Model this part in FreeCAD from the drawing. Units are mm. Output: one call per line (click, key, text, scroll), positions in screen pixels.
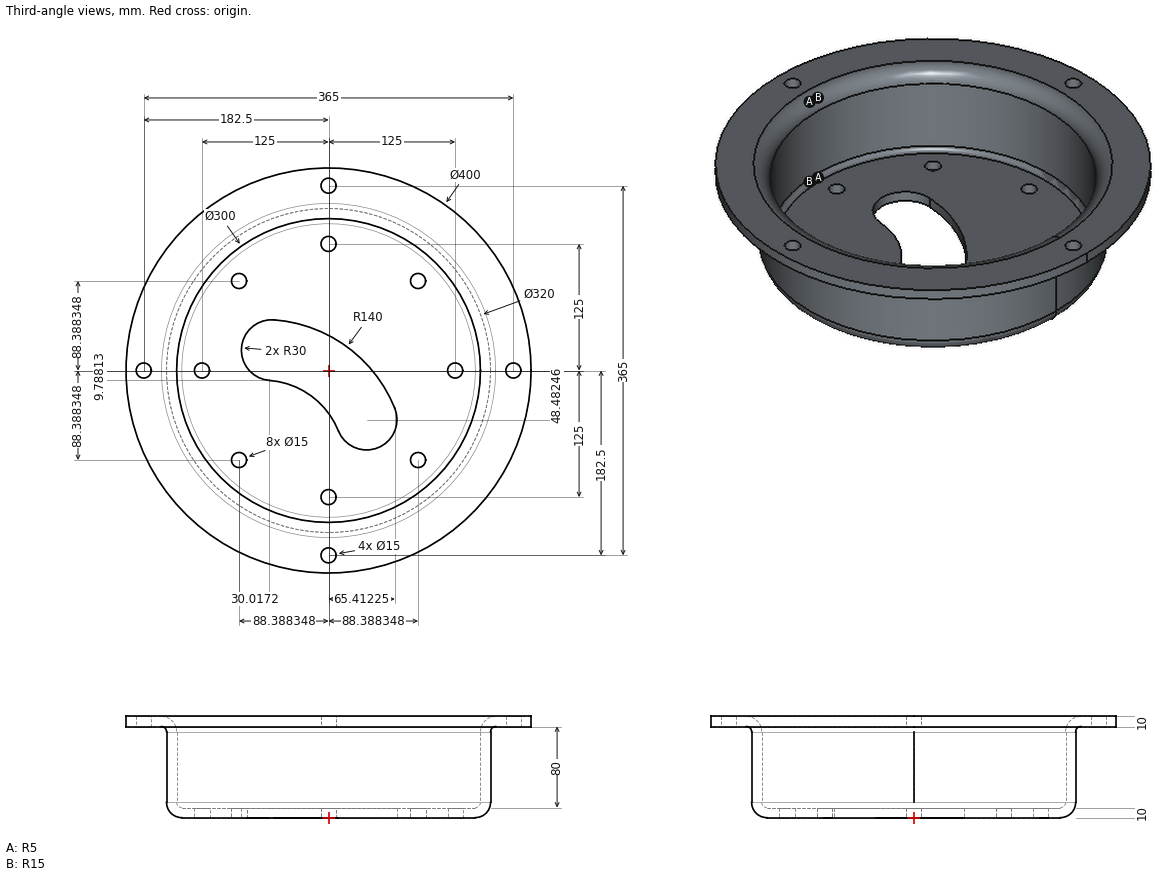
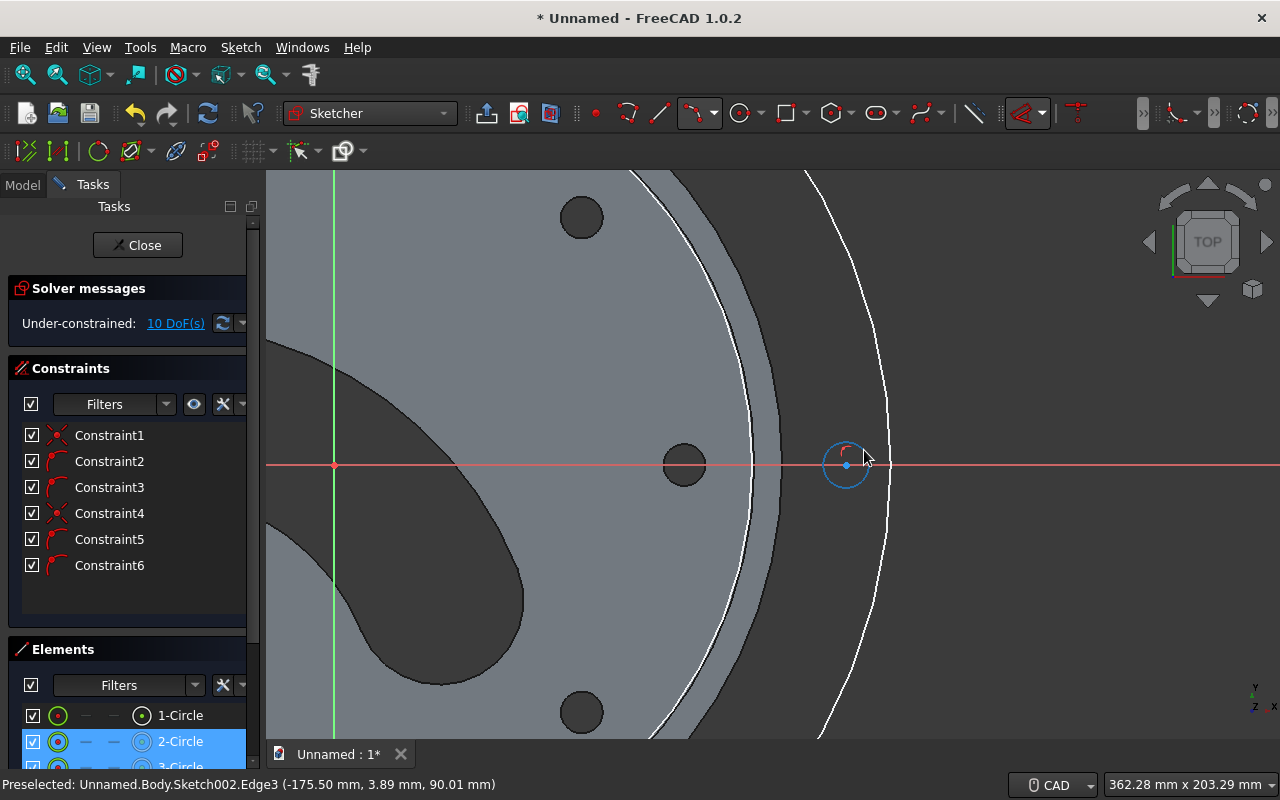
click(862, 449)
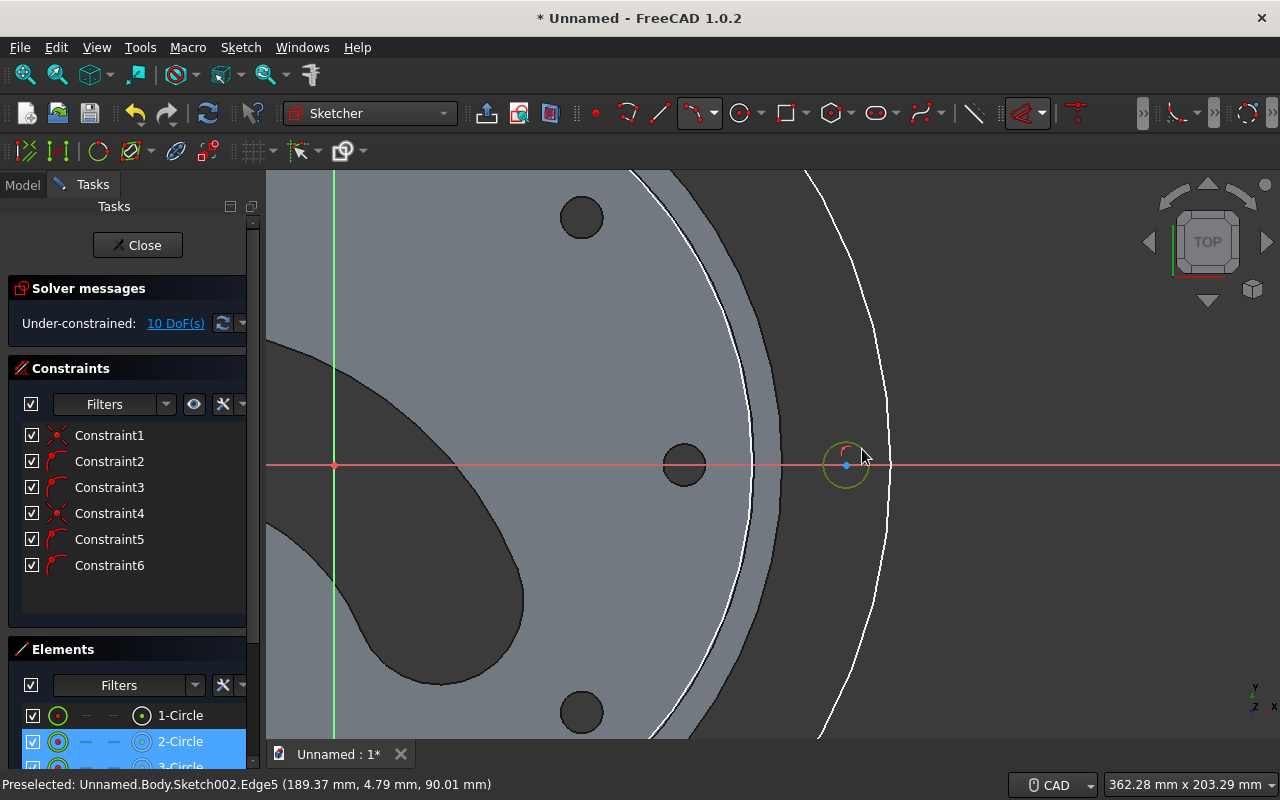
scroll(864, 450, down, 6)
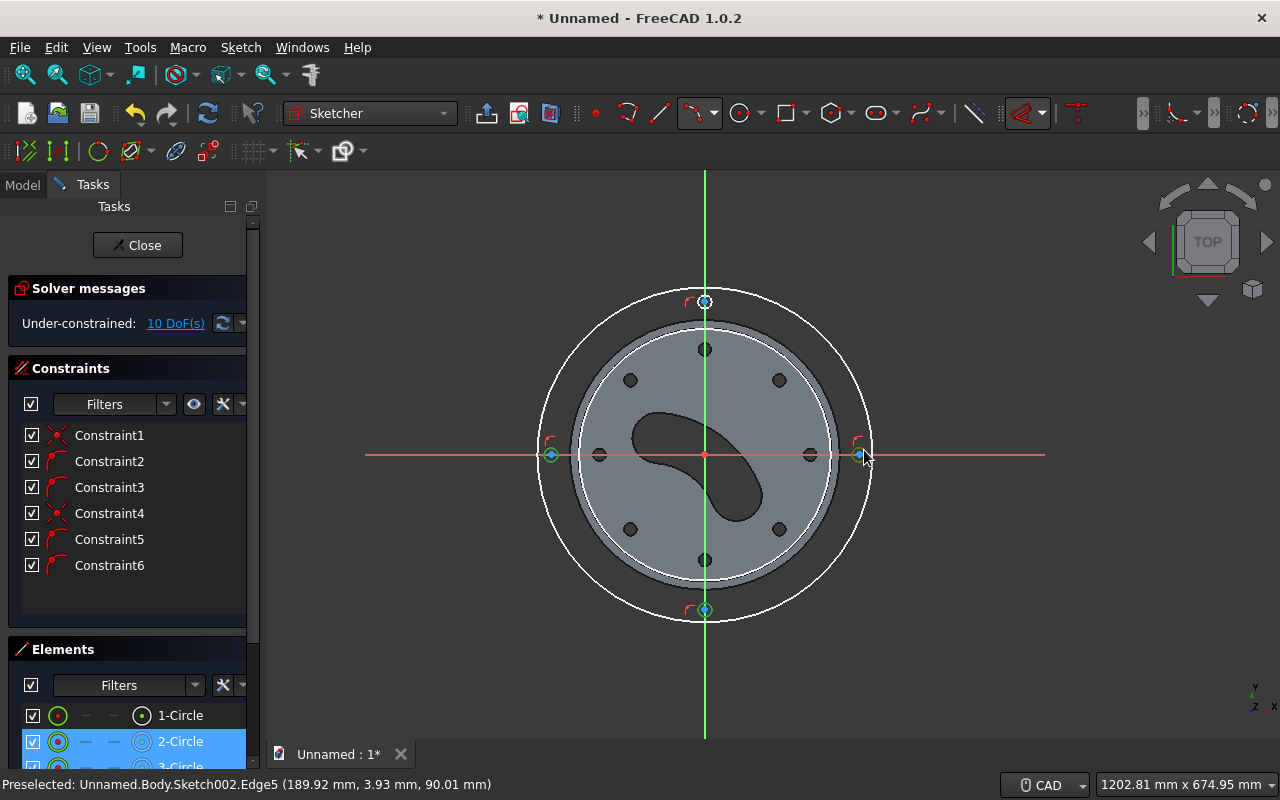
scroll(710, 297, up, 6)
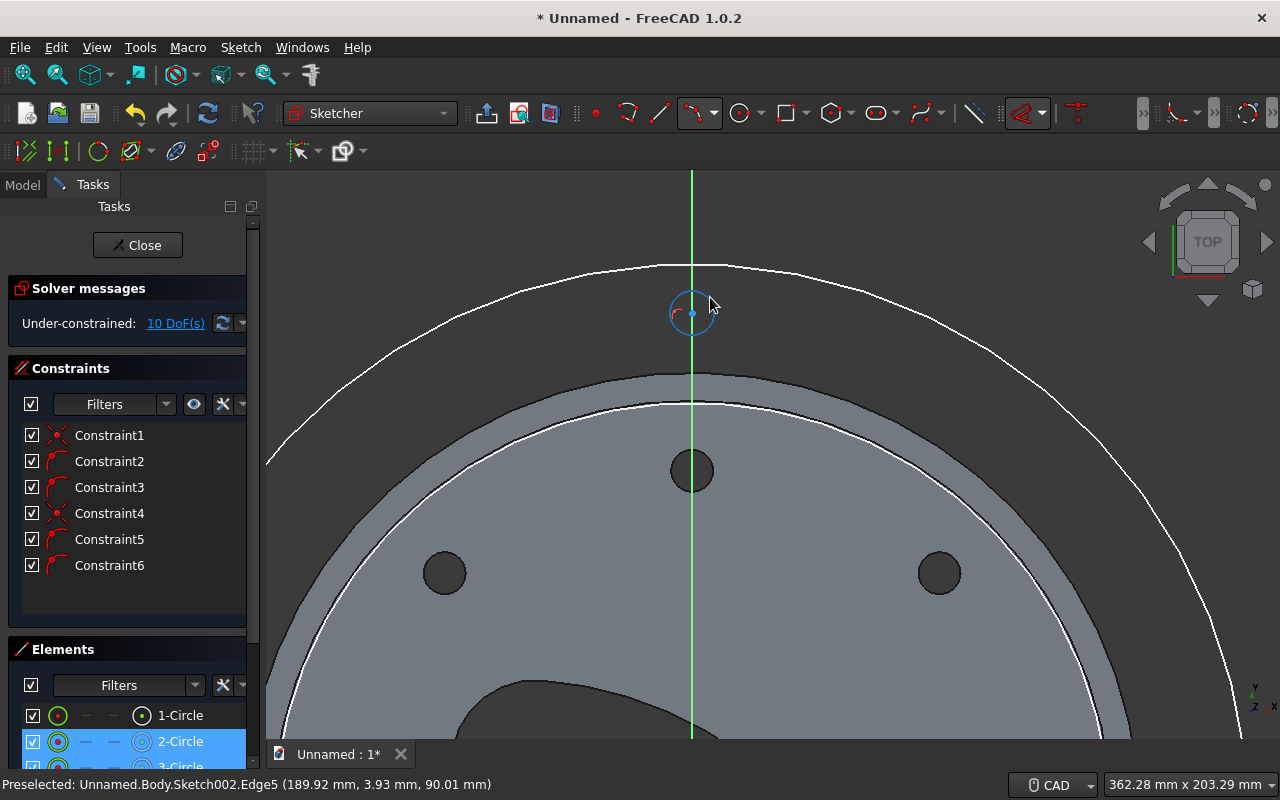
click(708, 297)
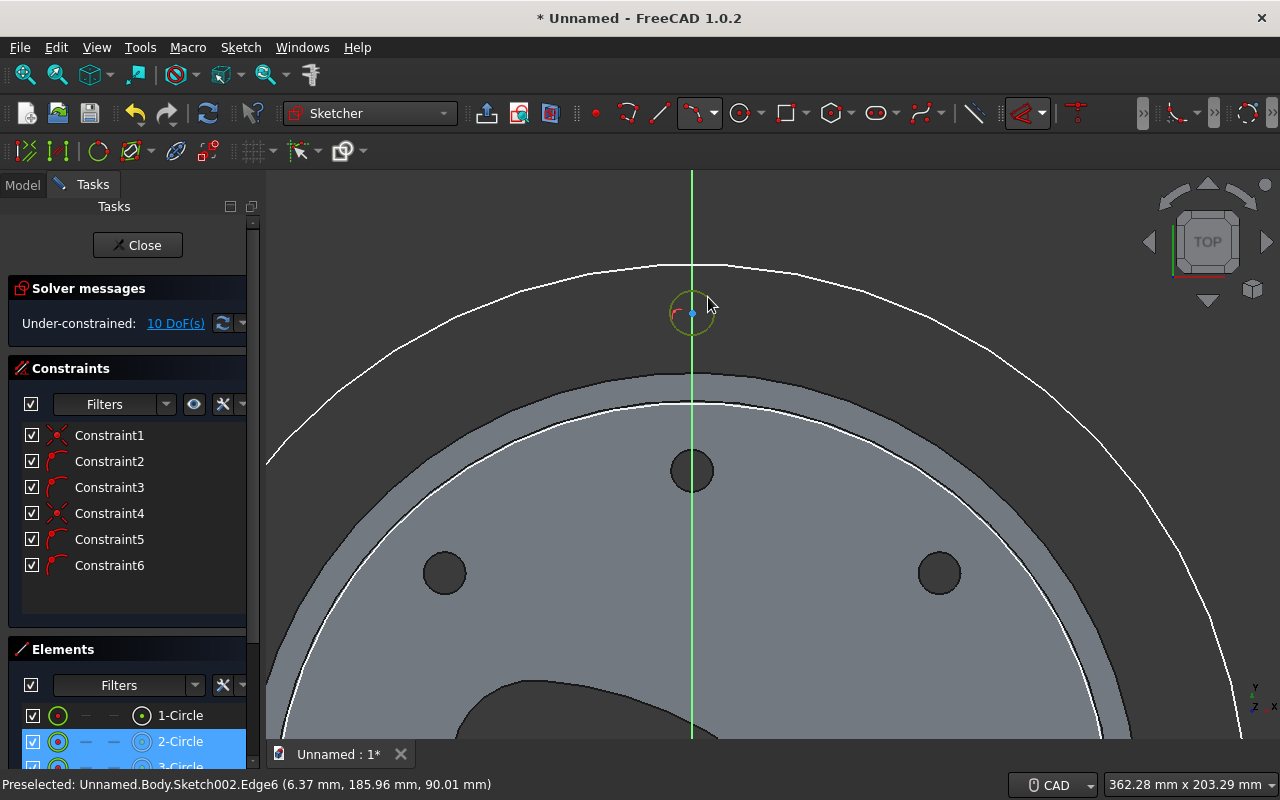
key(e)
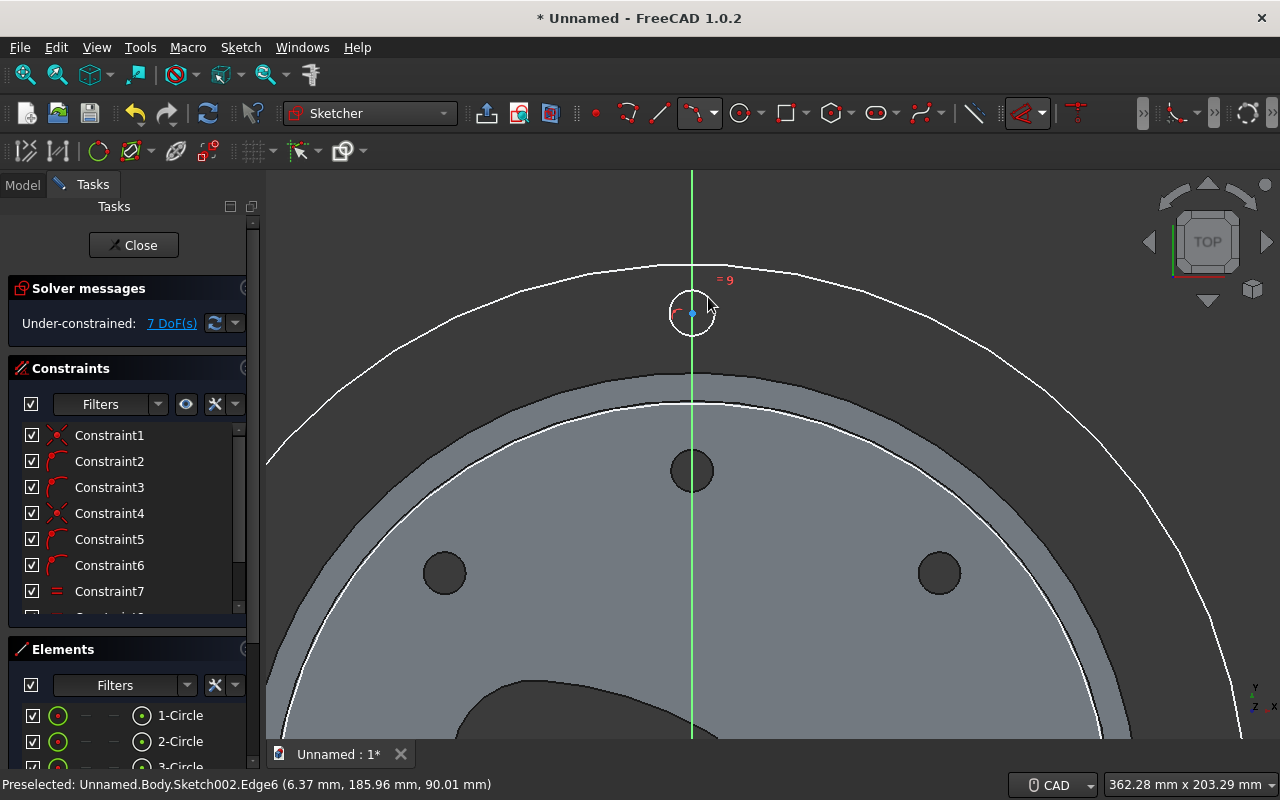
click(1084, 426)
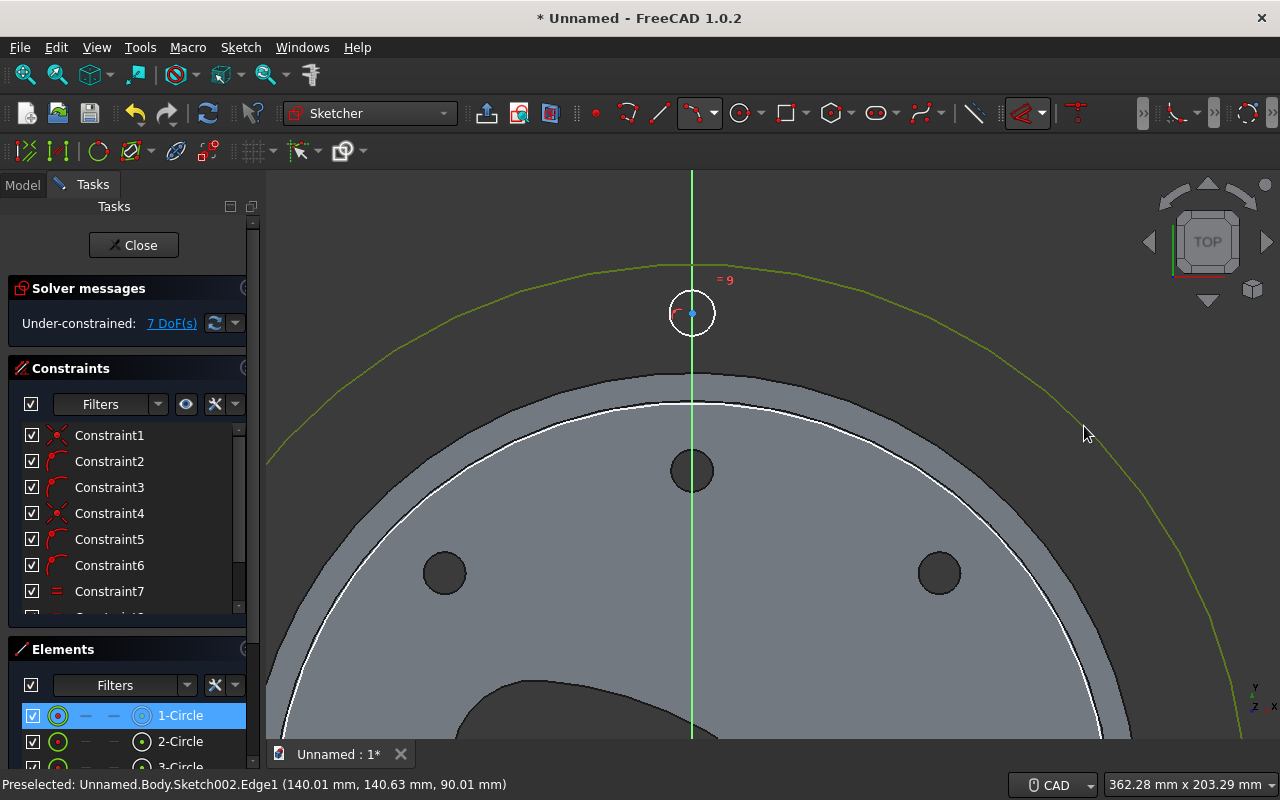
click(1044, 114)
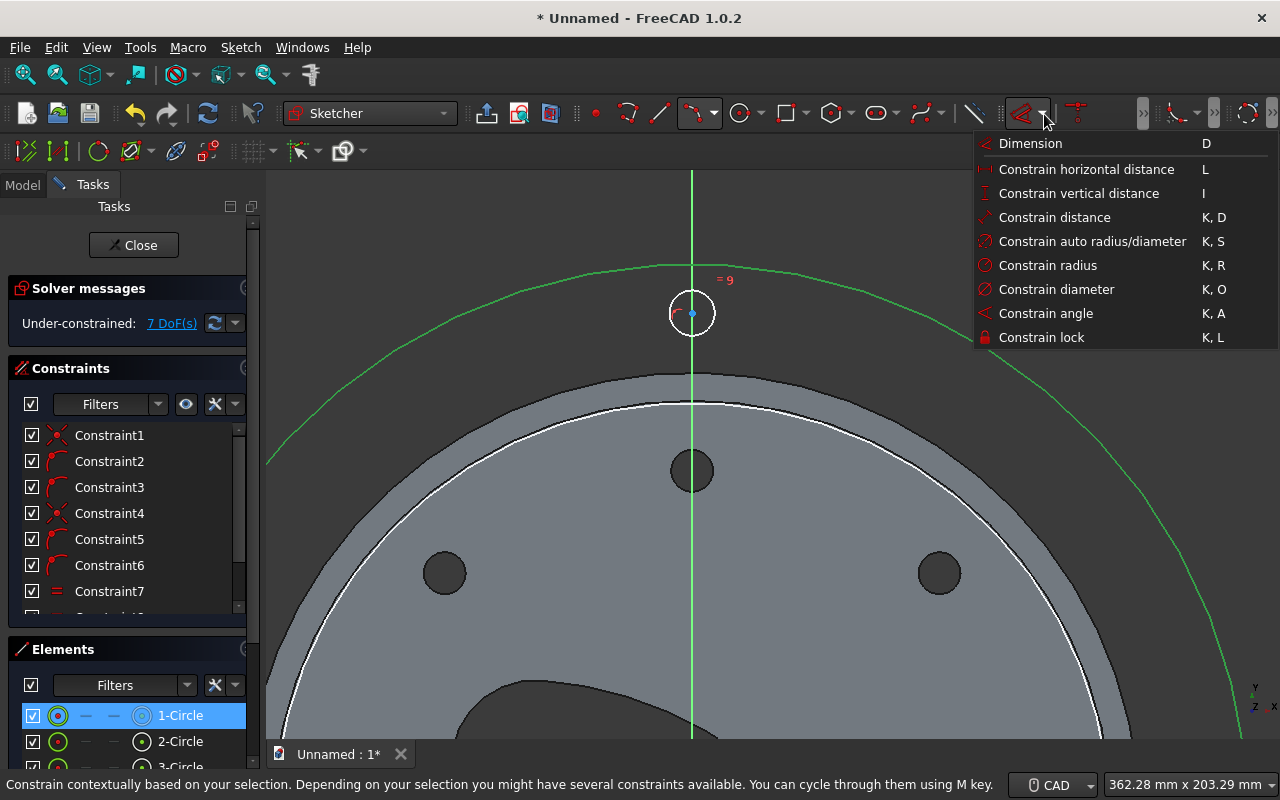
click(1126, 289)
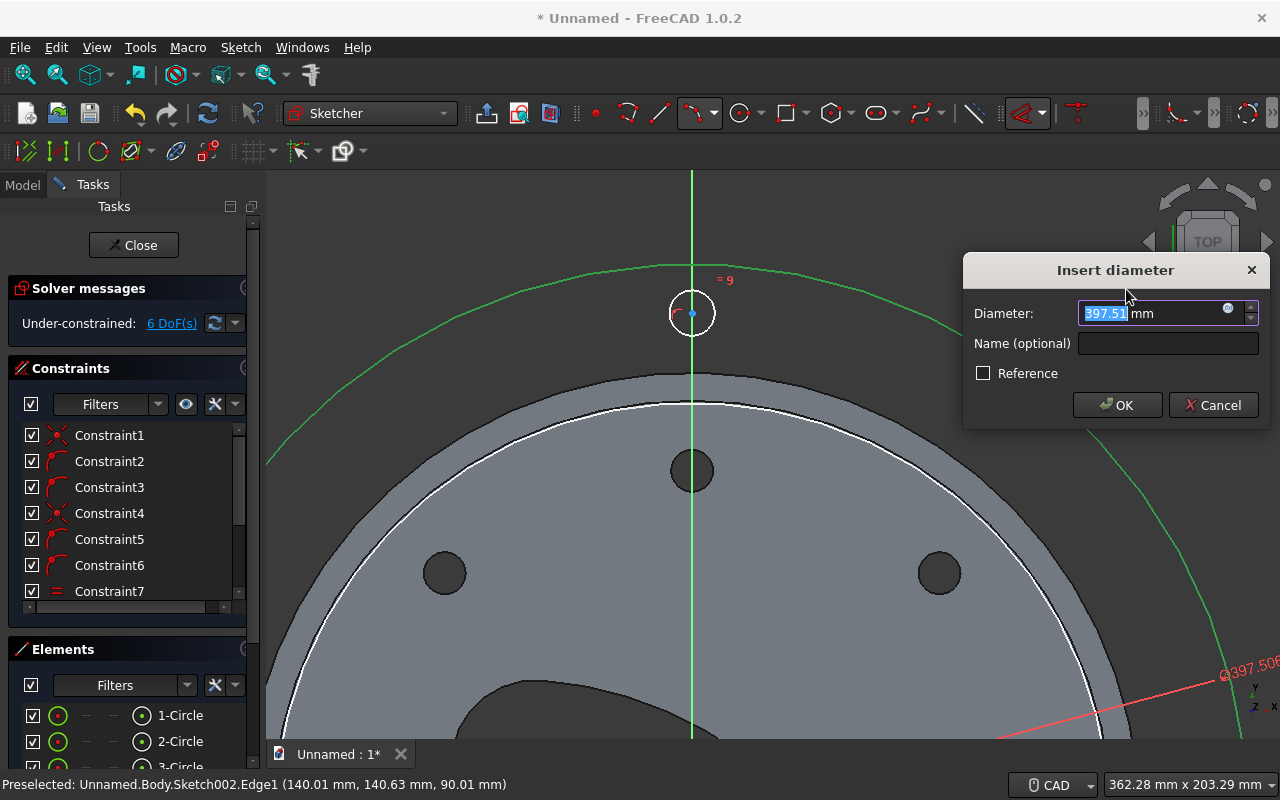
text(400)
key(Return)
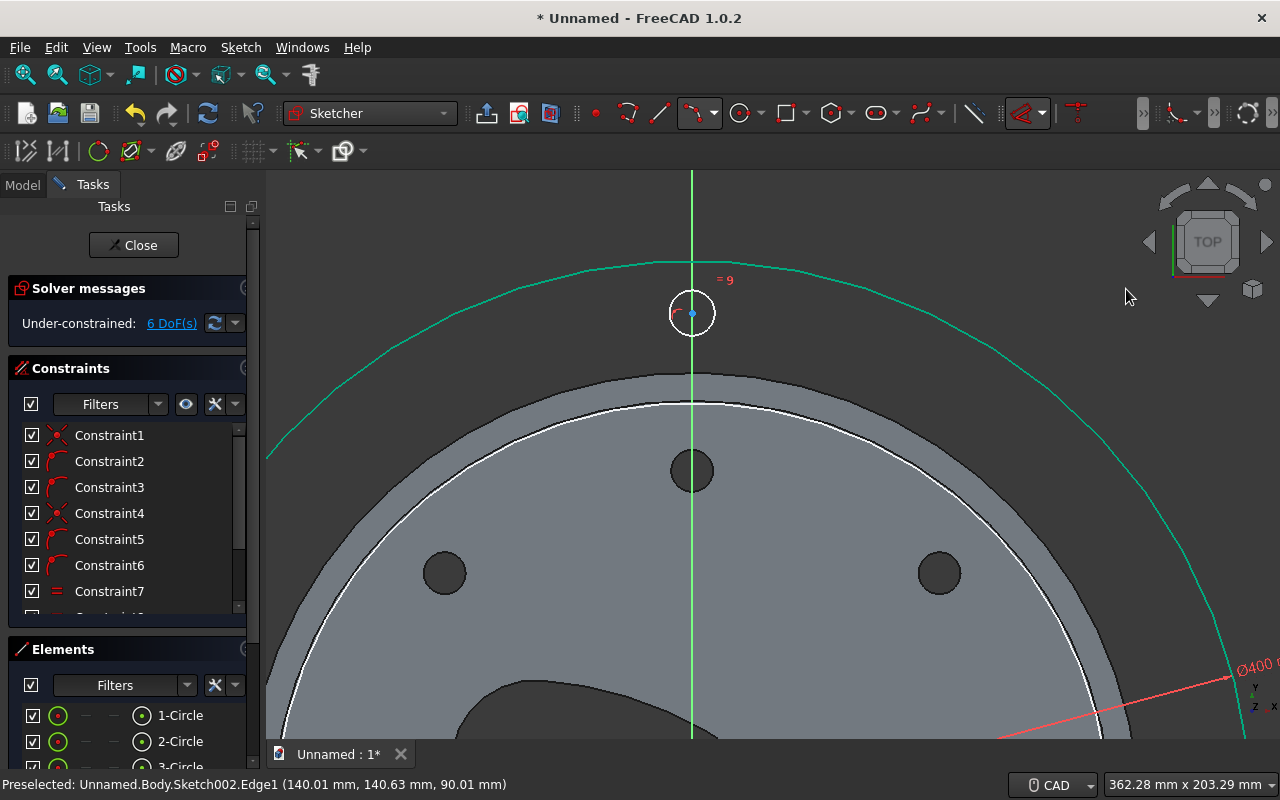
scroll(710, 297, down, 6)